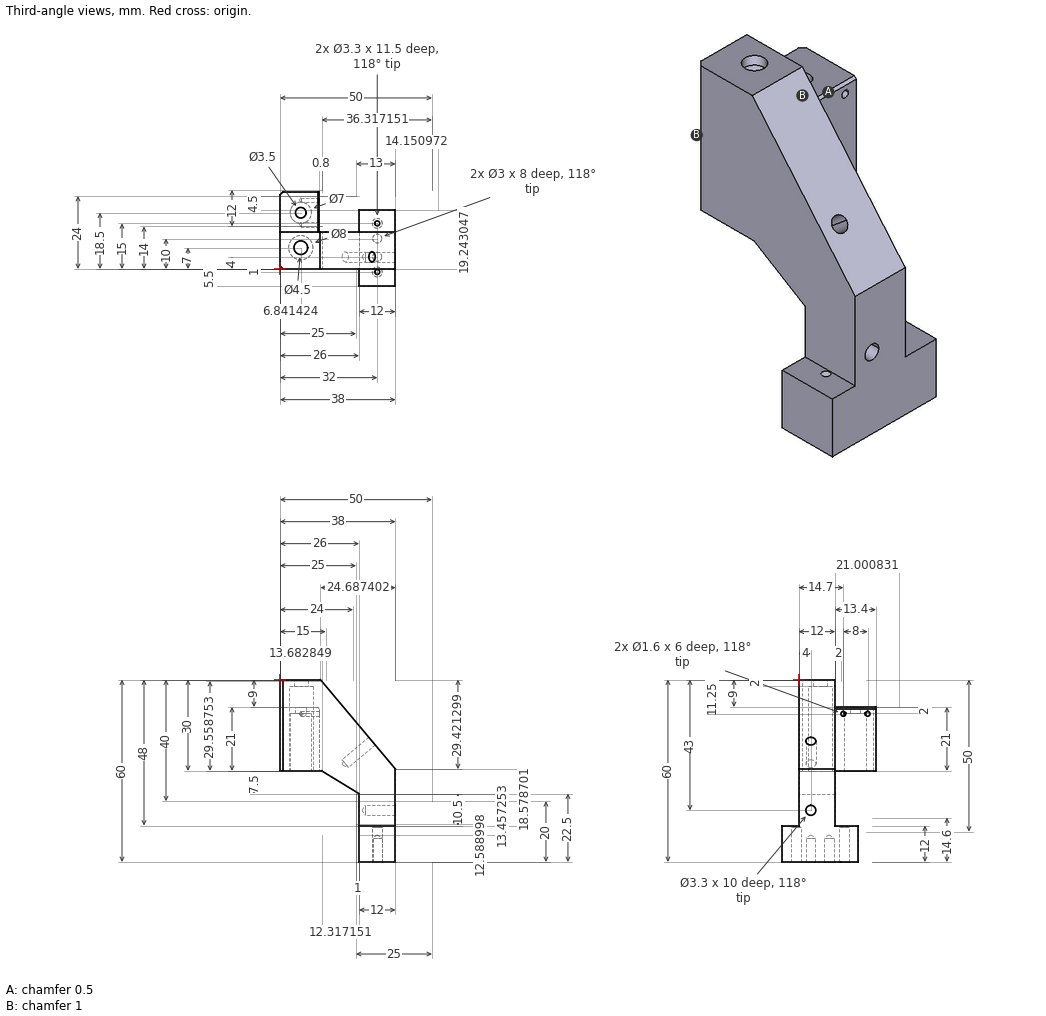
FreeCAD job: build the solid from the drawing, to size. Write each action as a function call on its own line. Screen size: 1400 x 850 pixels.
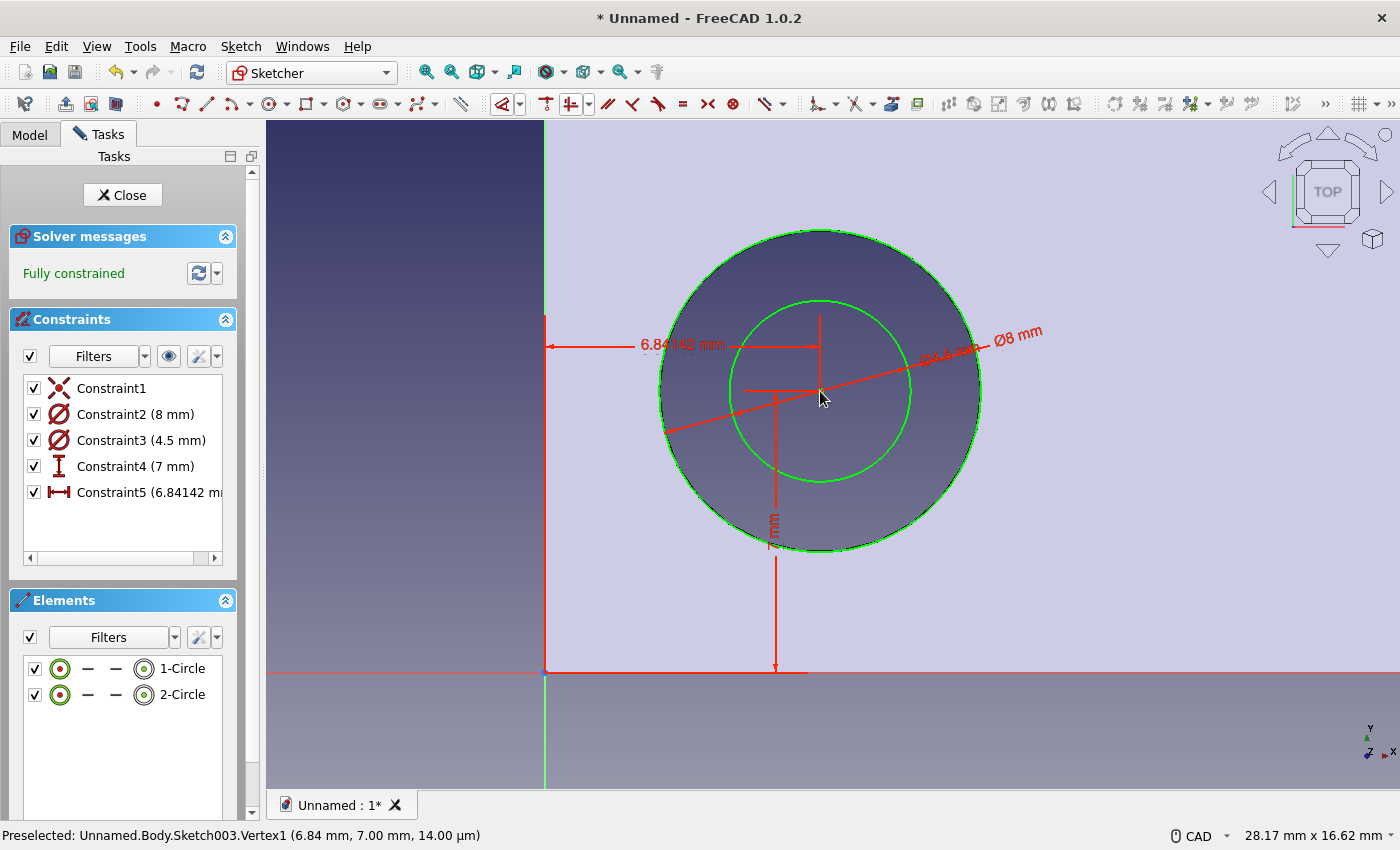
click(123, 195)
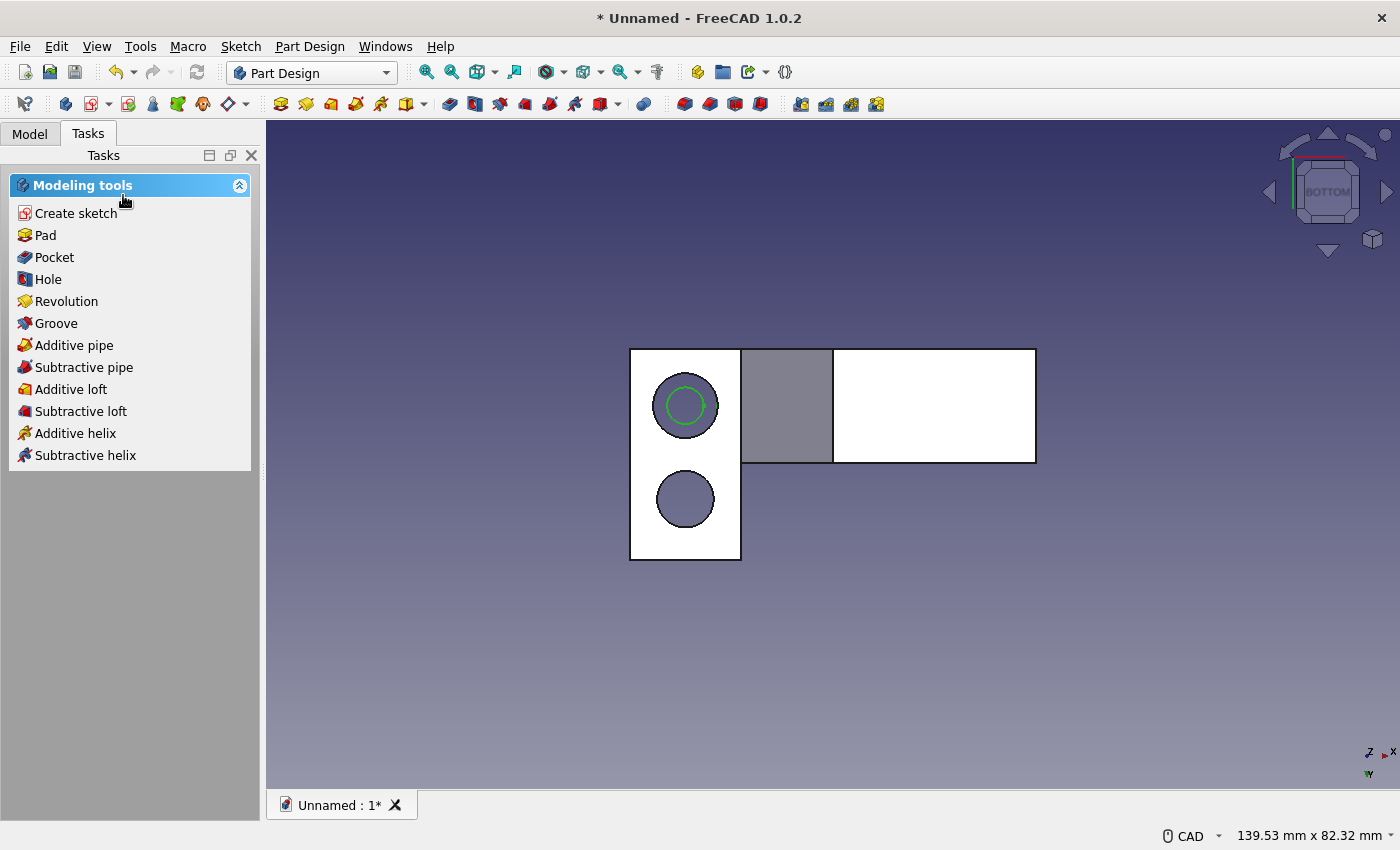
click(281, 104)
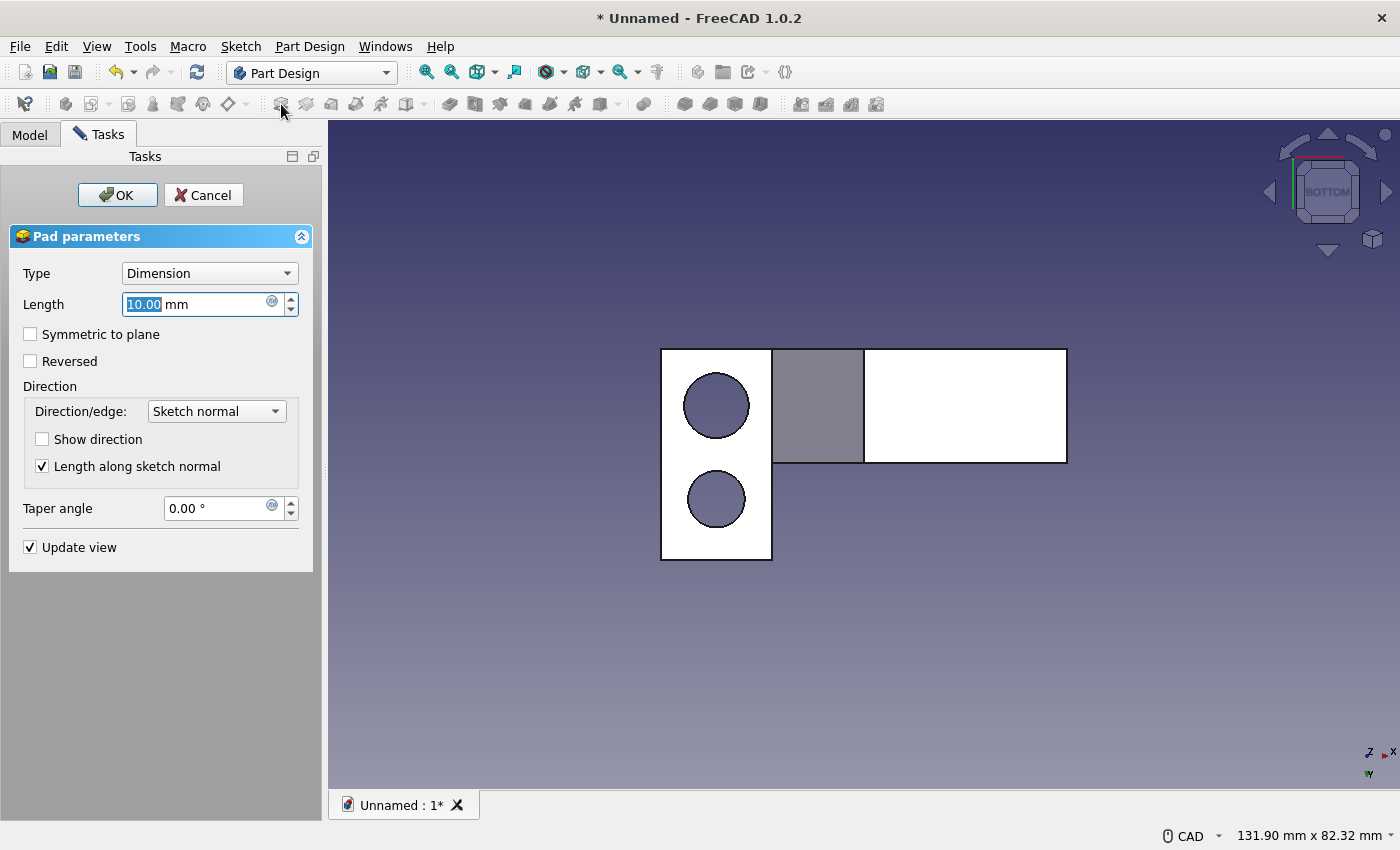
text(2)
key(Tab)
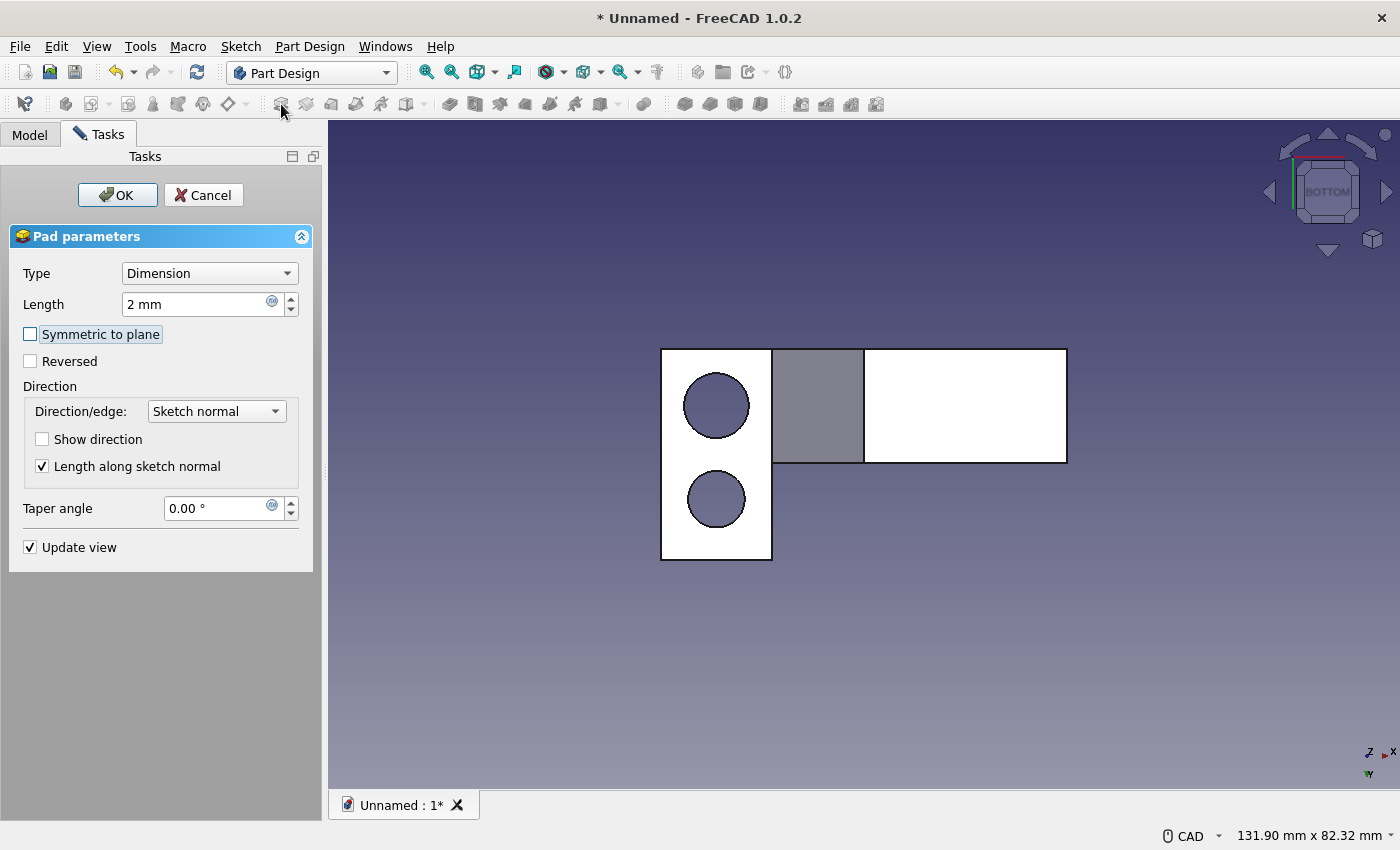
click(31, 361)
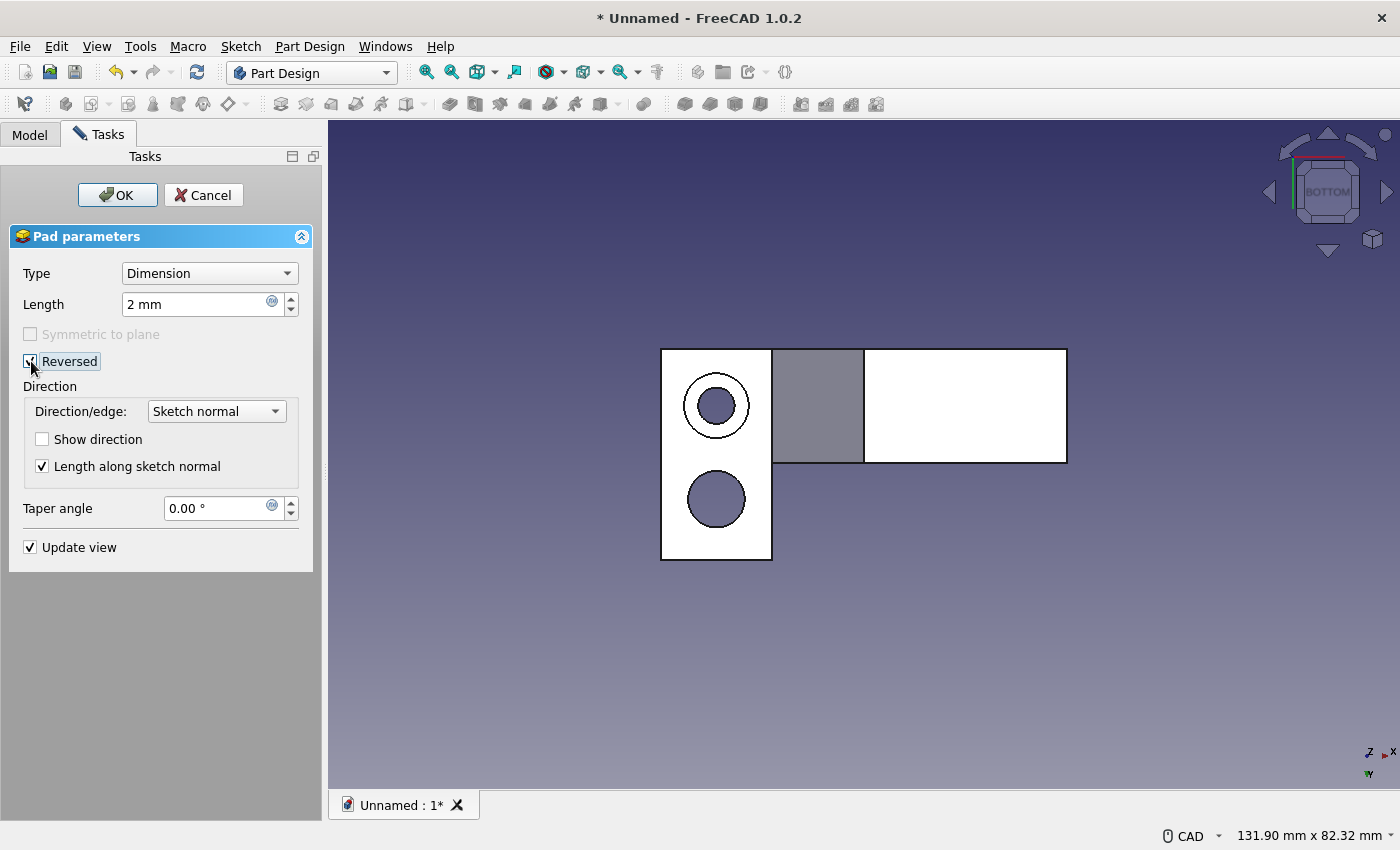
click(118, 195)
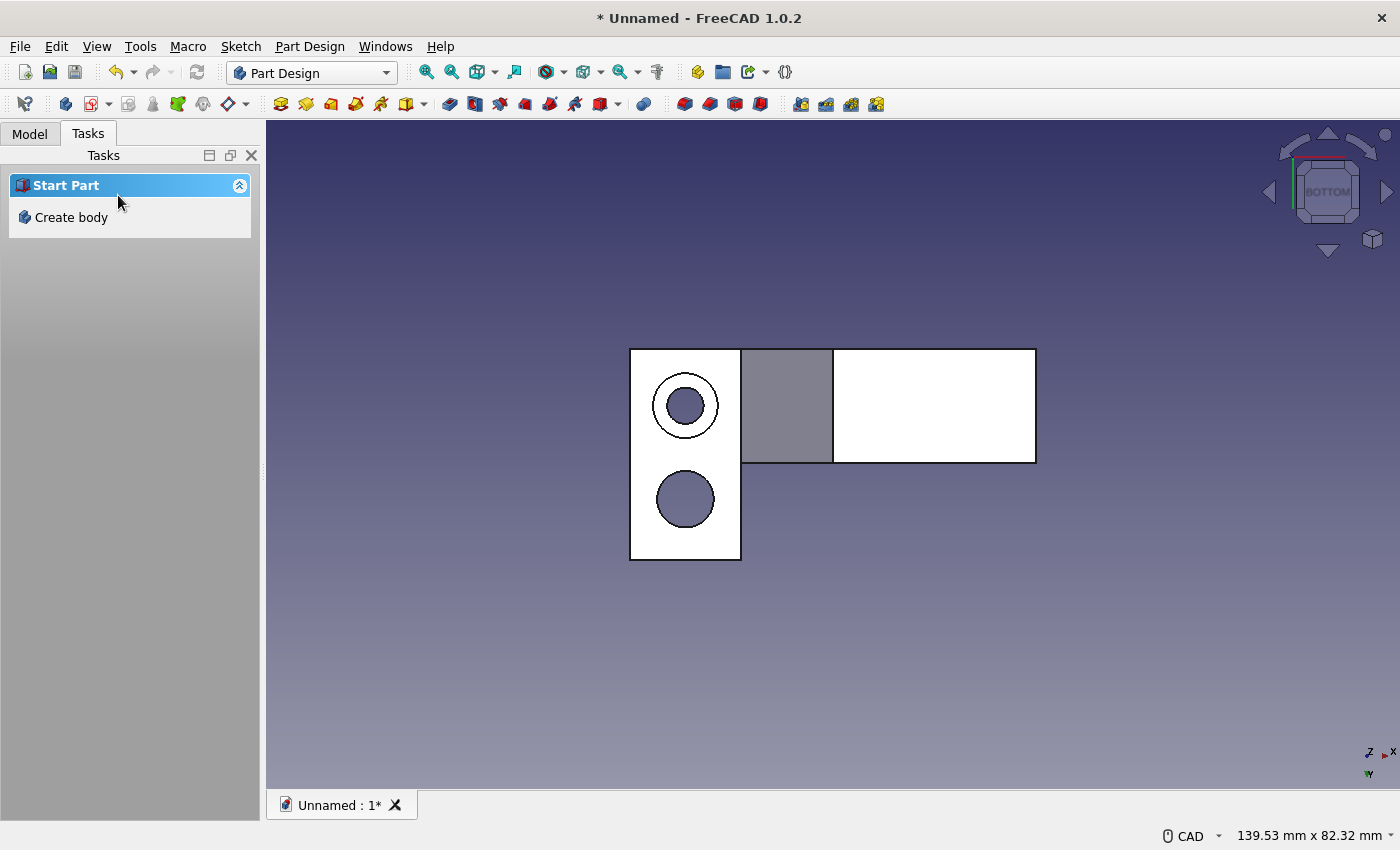
click(427, 72)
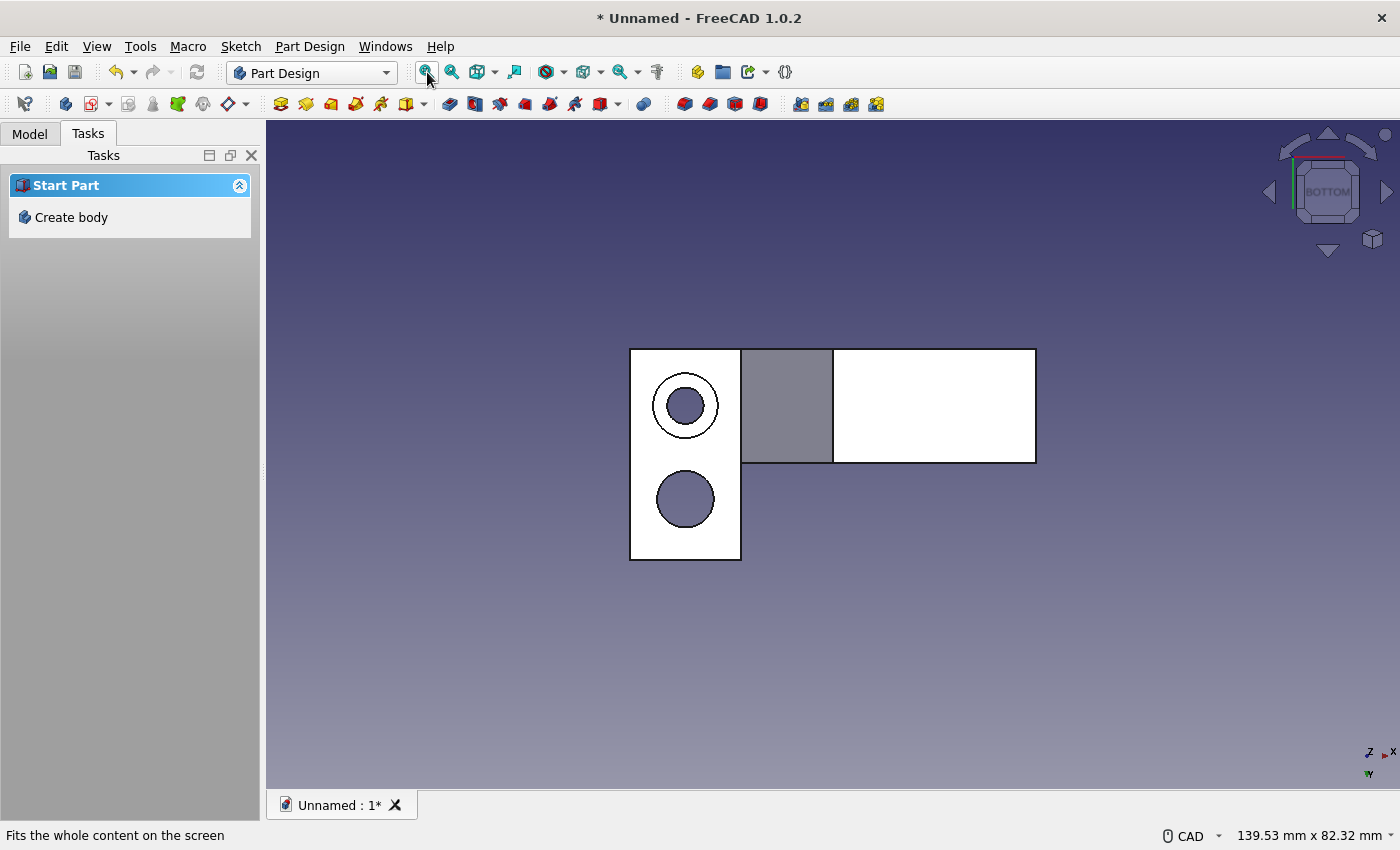
click(90, 104)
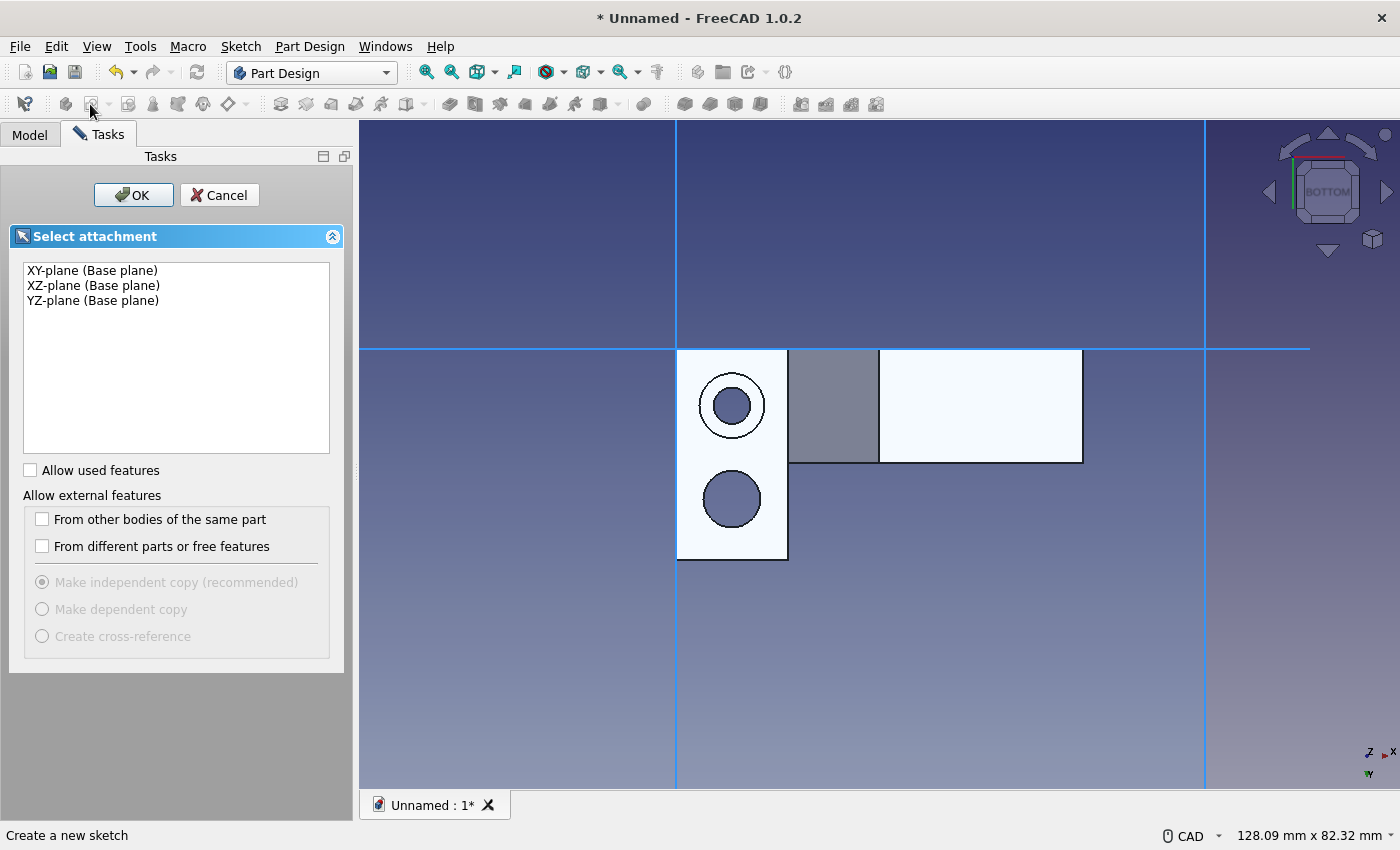
click(84, 300)